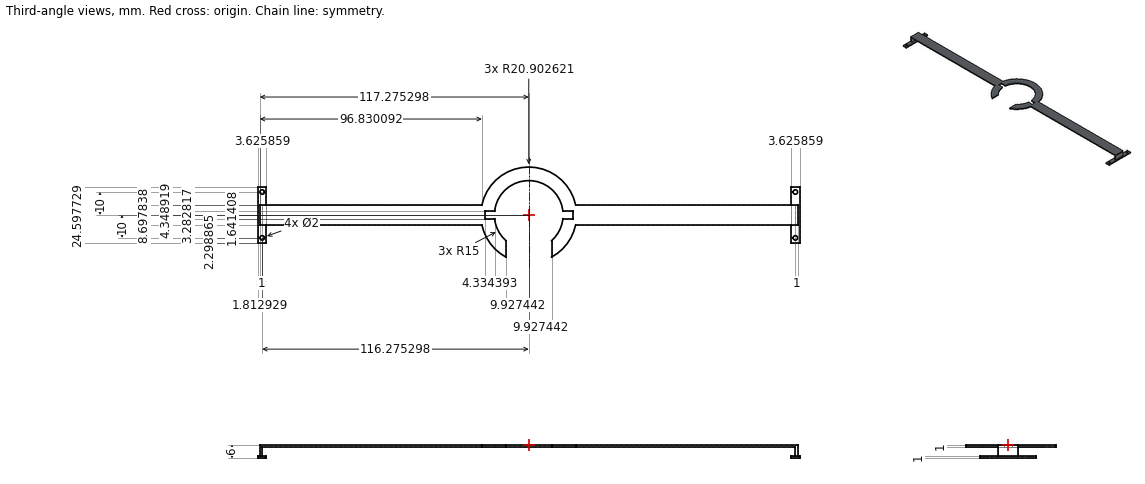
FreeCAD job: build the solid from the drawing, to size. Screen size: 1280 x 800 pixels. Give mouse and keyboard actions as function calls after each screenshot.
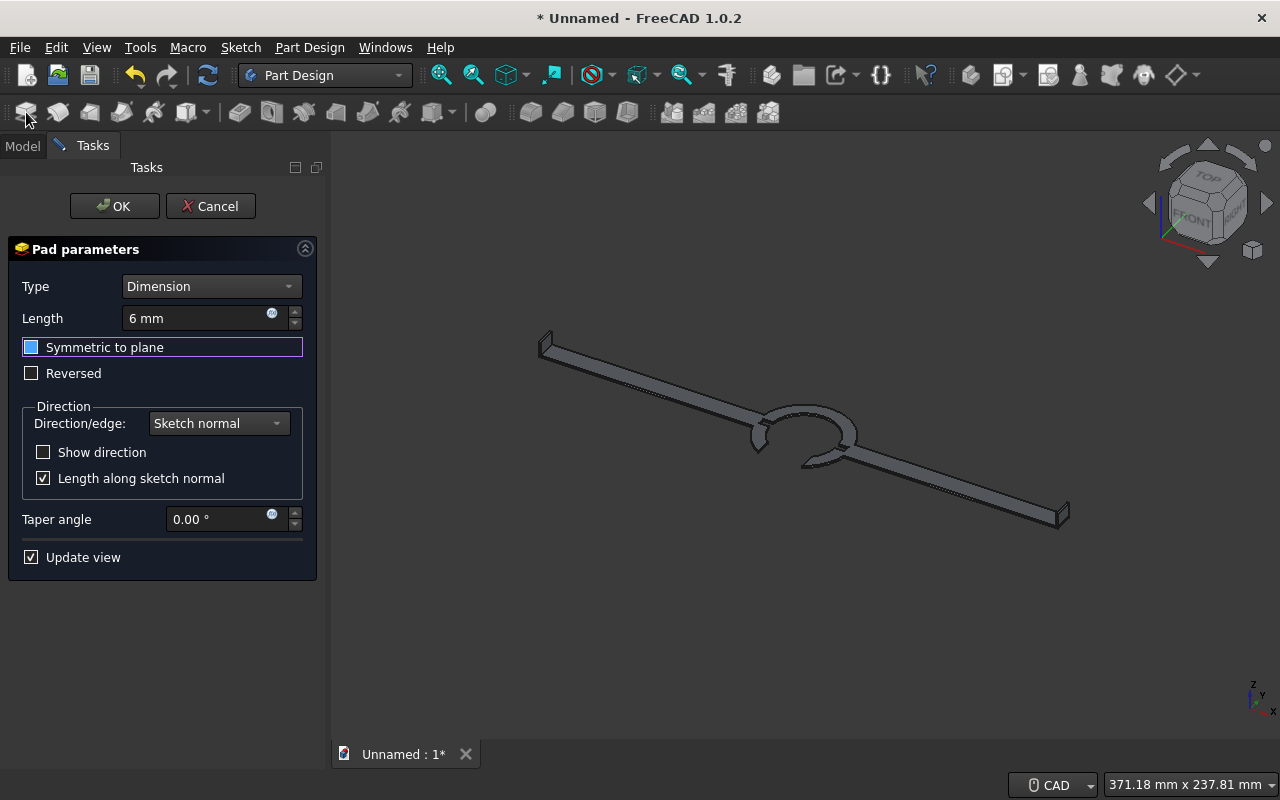
click(30, 373)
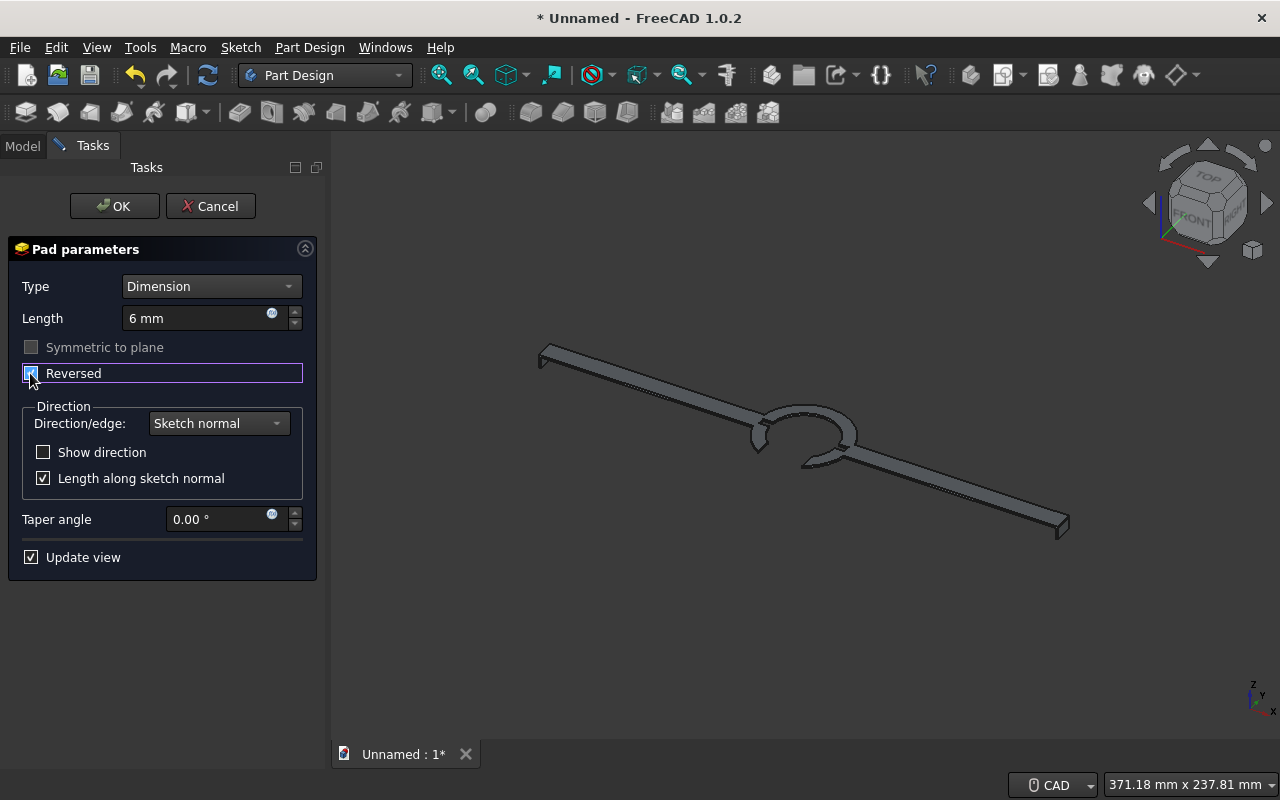
click(115, 206)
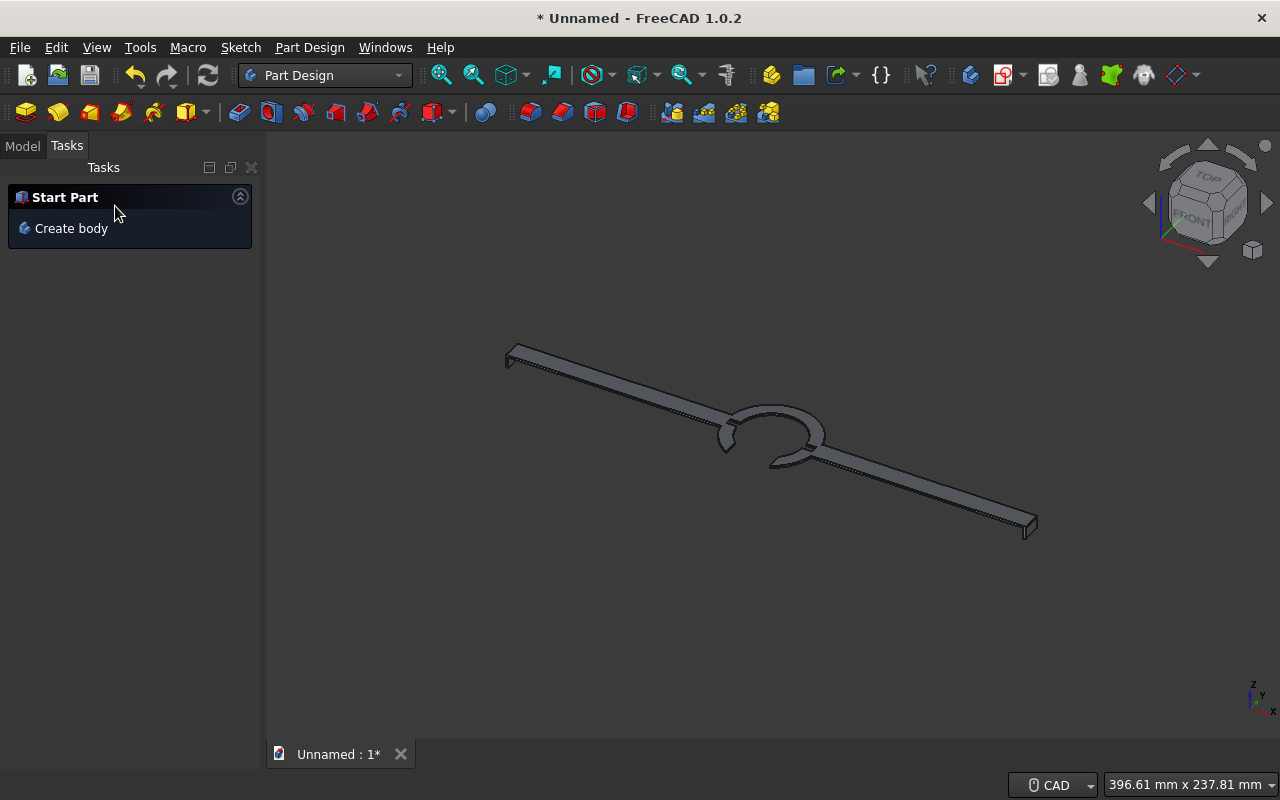
key(5)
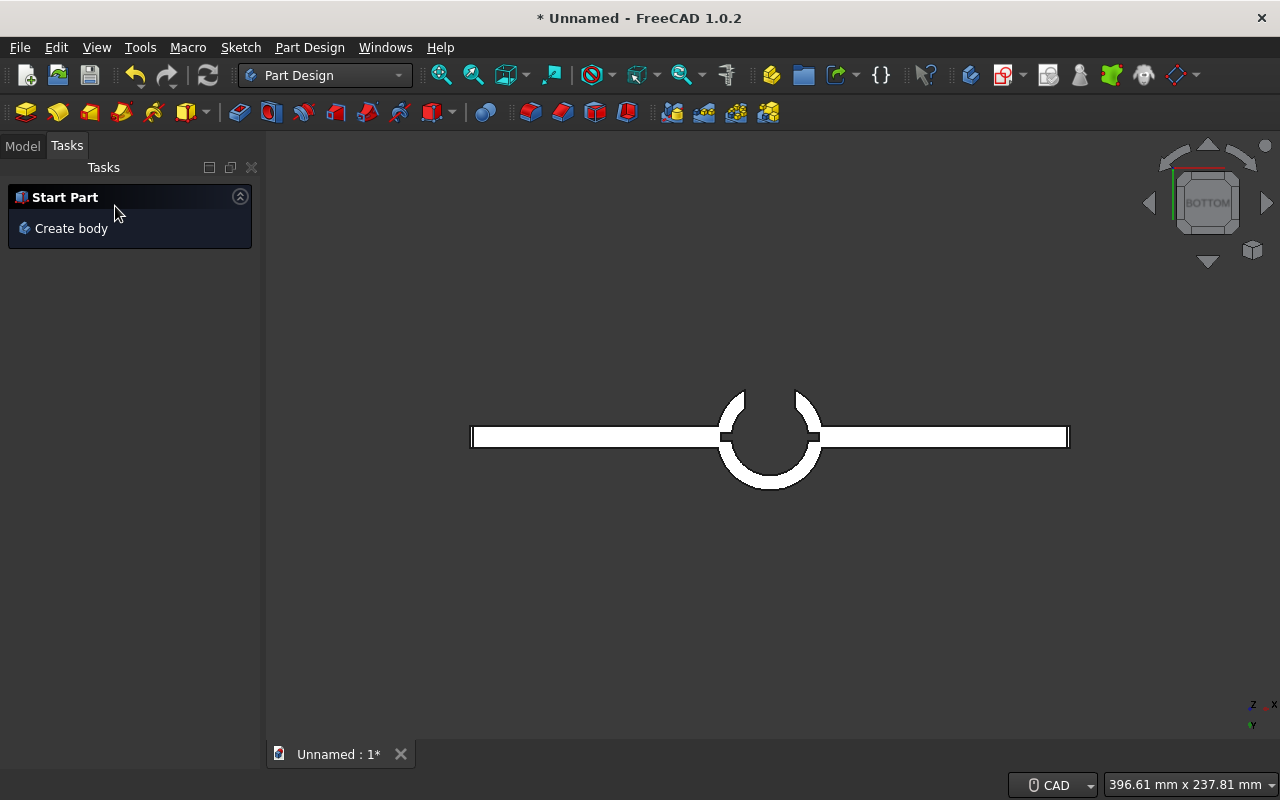
scroll(1069, 446, up, 12)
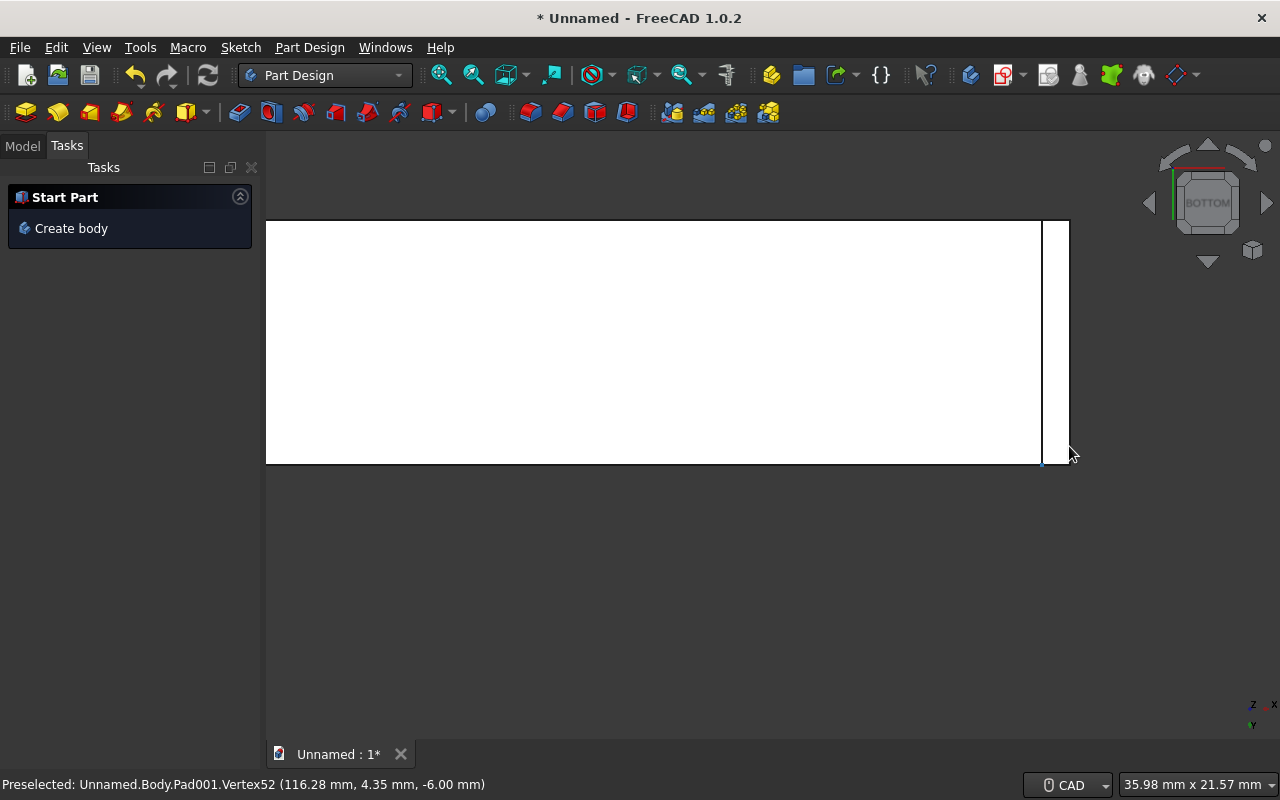
click(1056, 447)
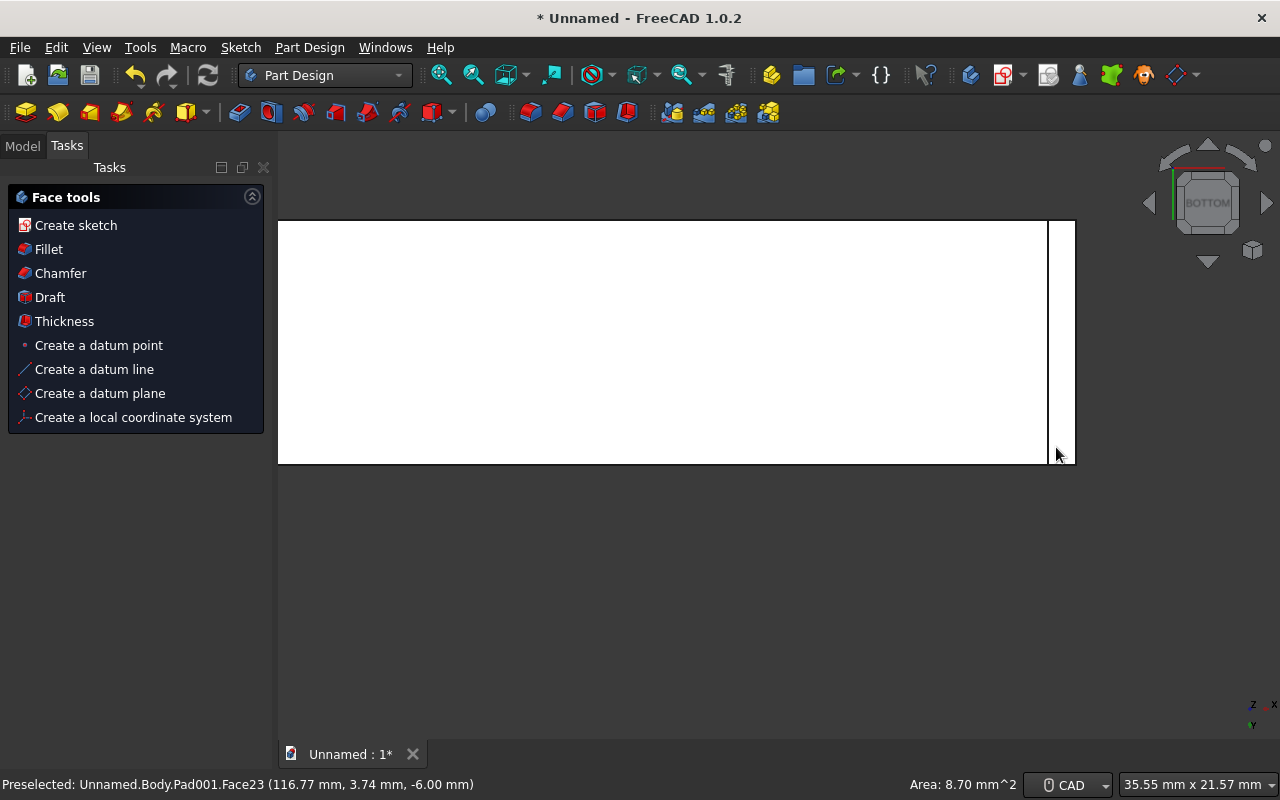
click(1004, 76)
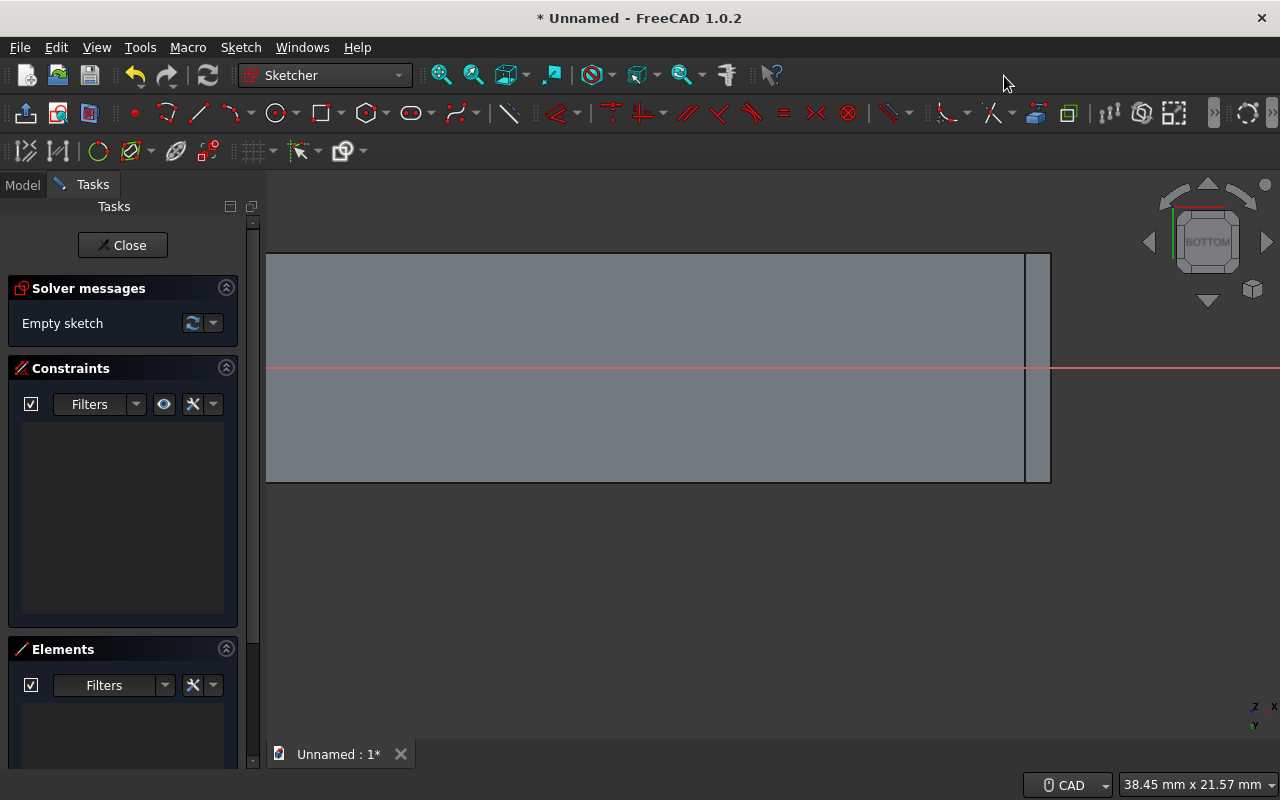
scroll(979, 463, down, 12)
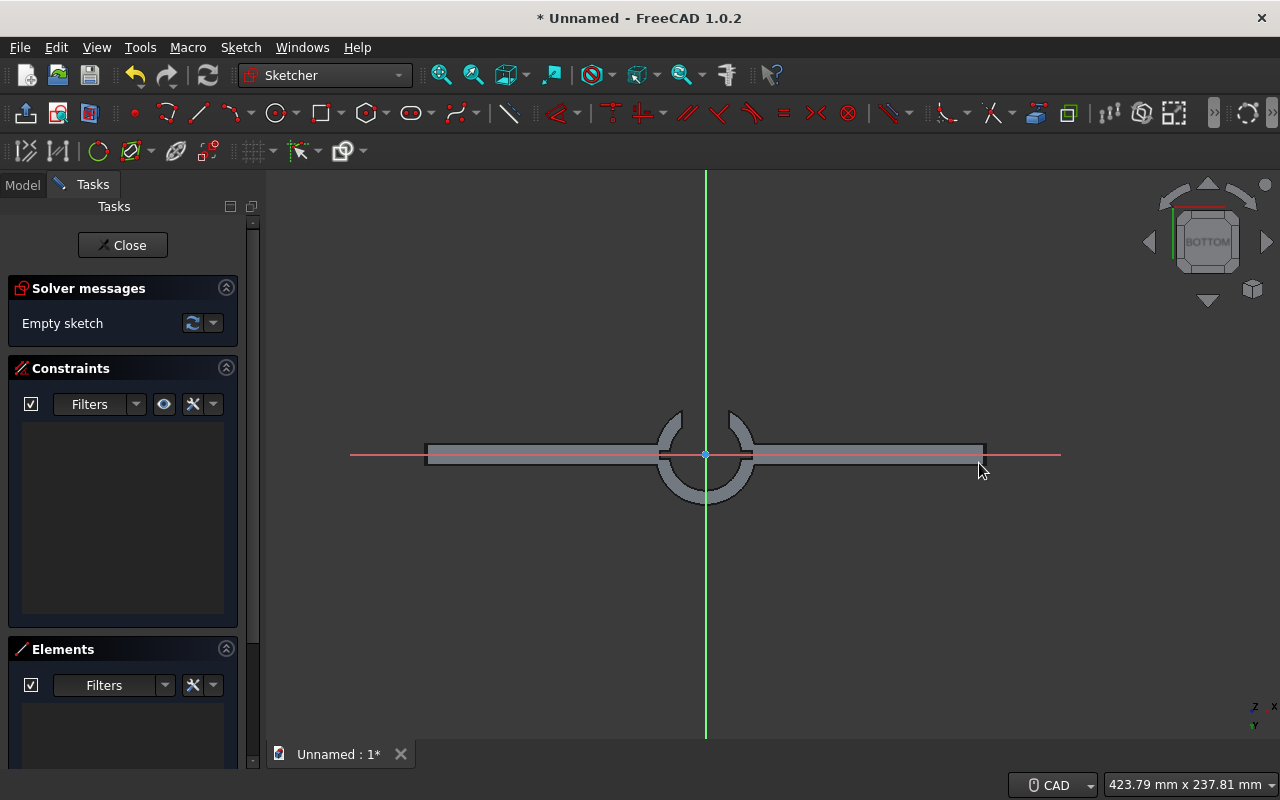
click(322, 114)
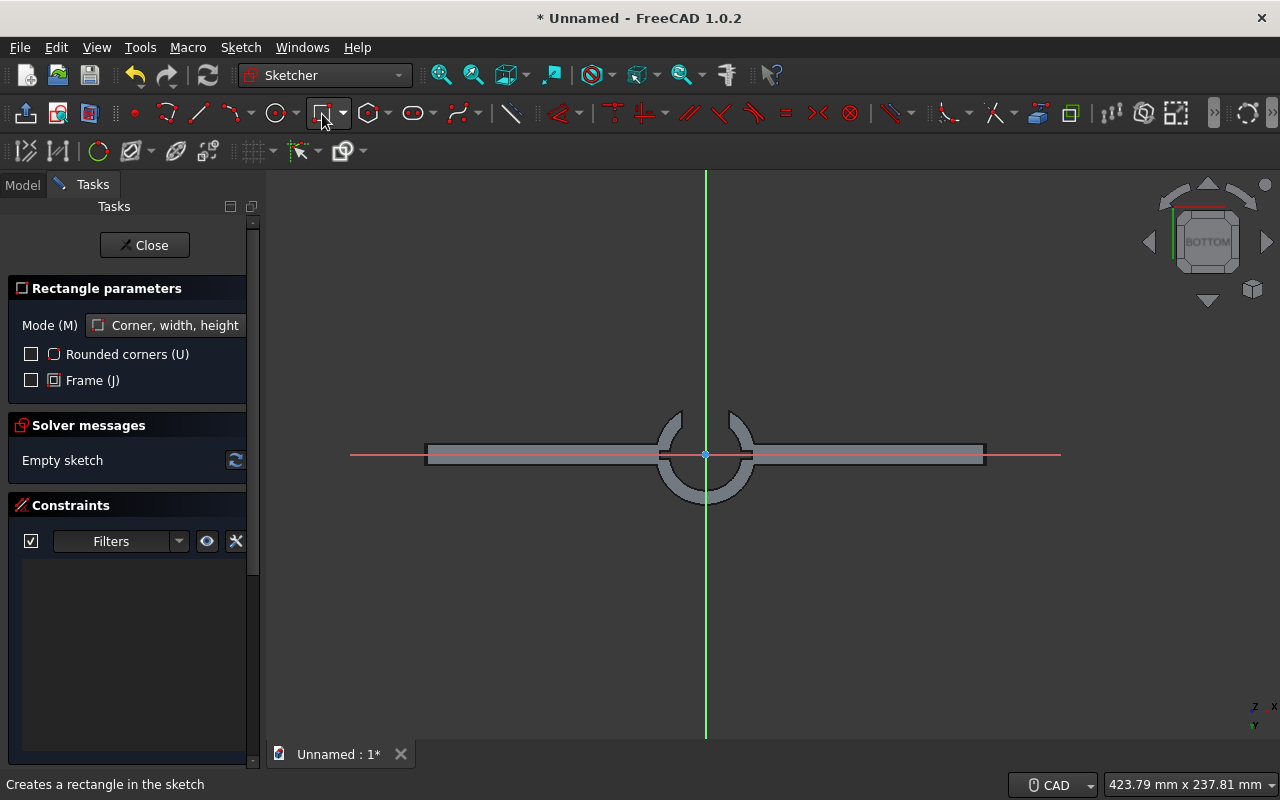
scroll(423, 425, up, 4)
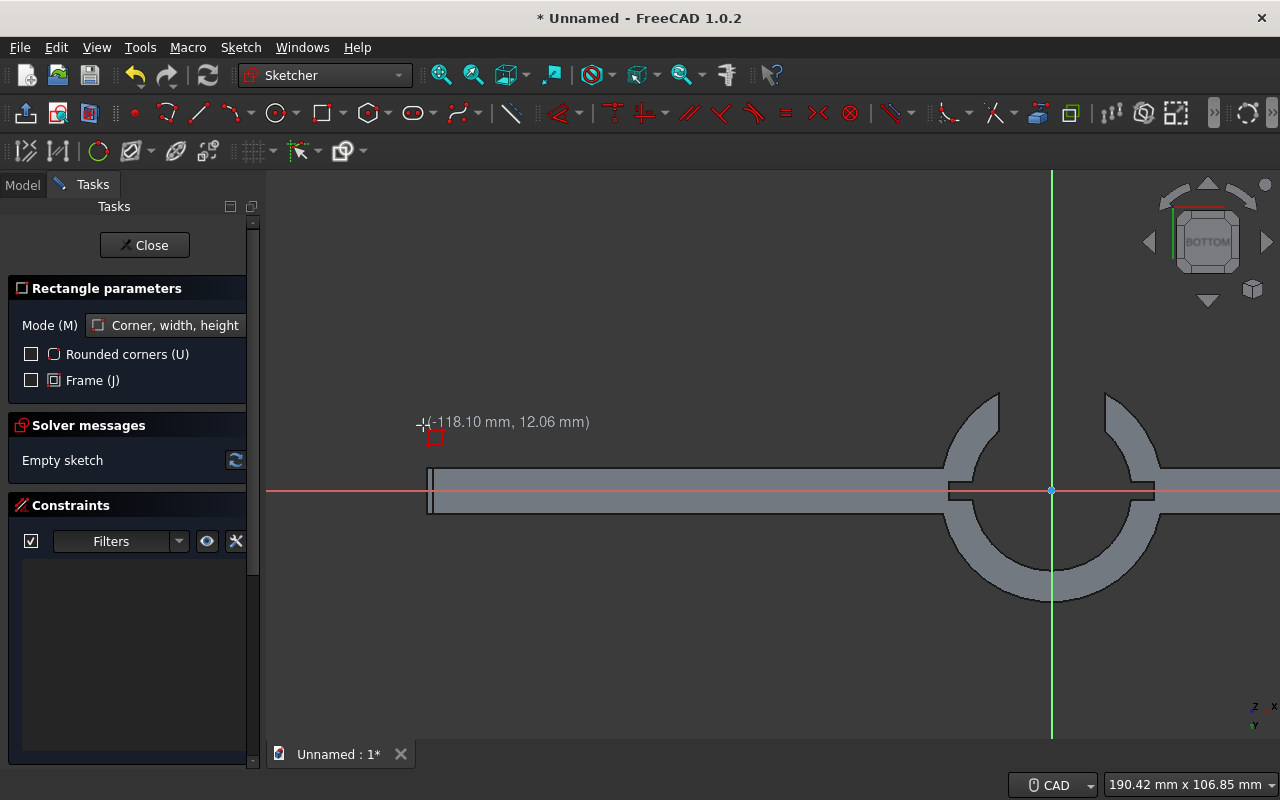
click(423, 425)
move(442, 556)